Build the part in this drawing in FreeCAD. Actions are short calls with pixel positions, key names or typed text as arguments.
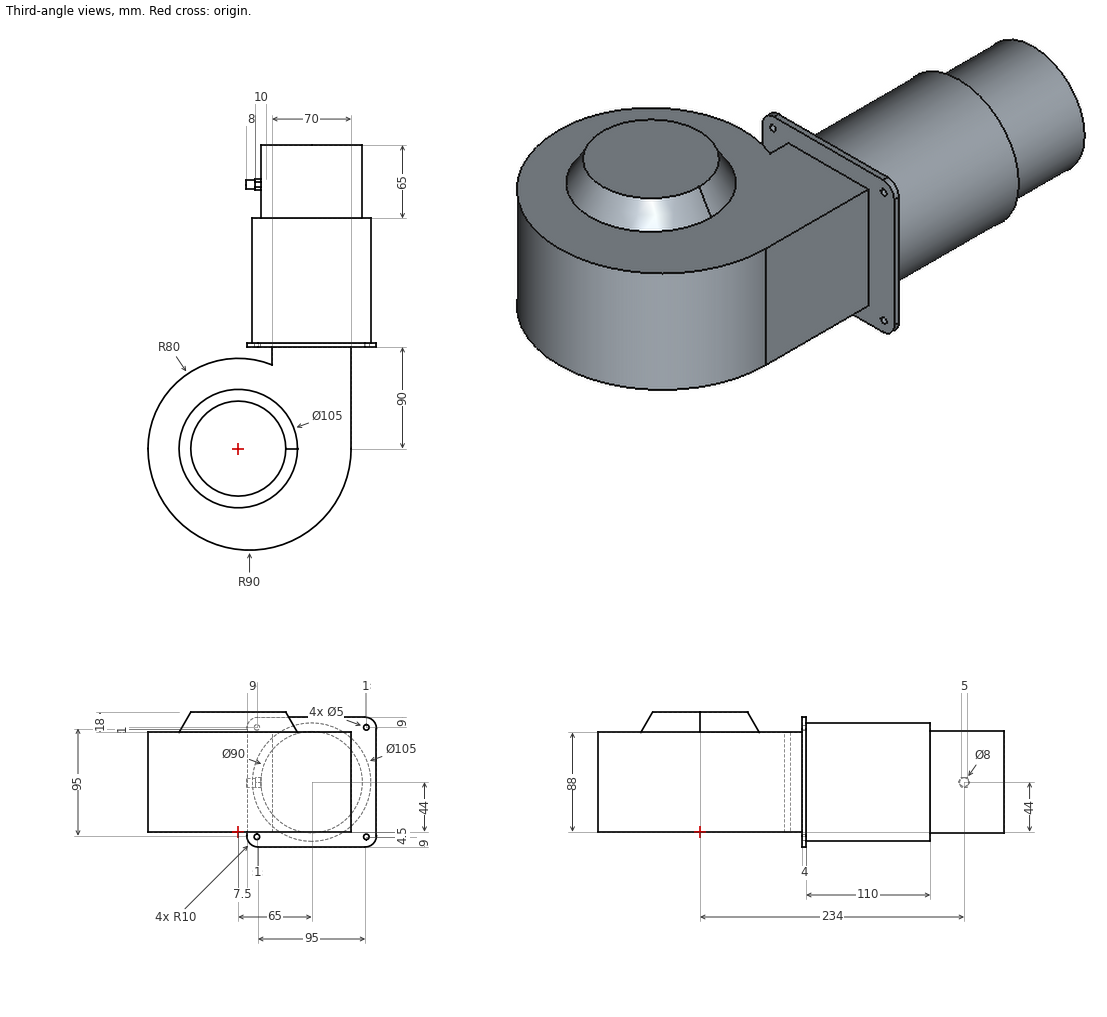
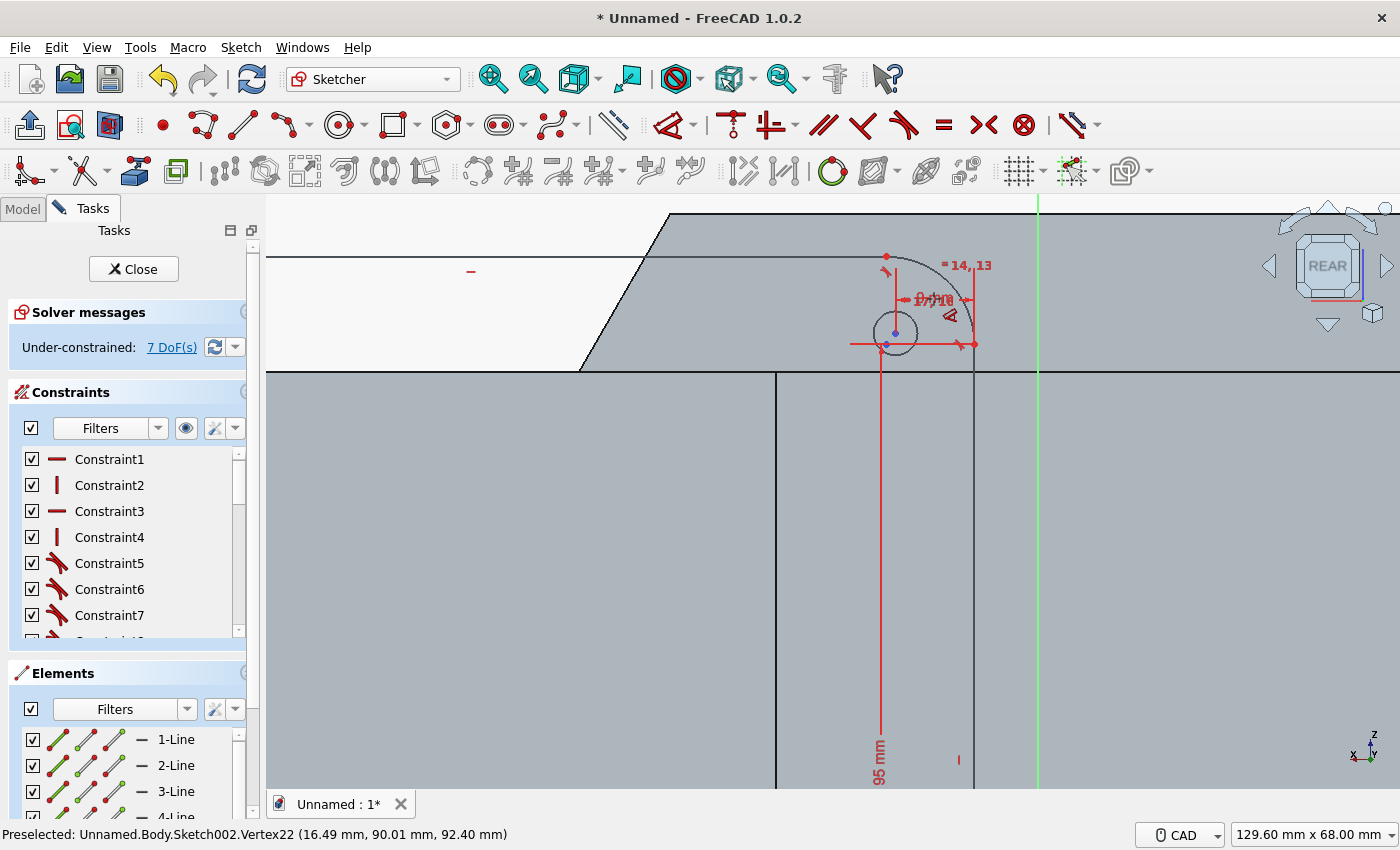
scroll(974, 344, up, 8)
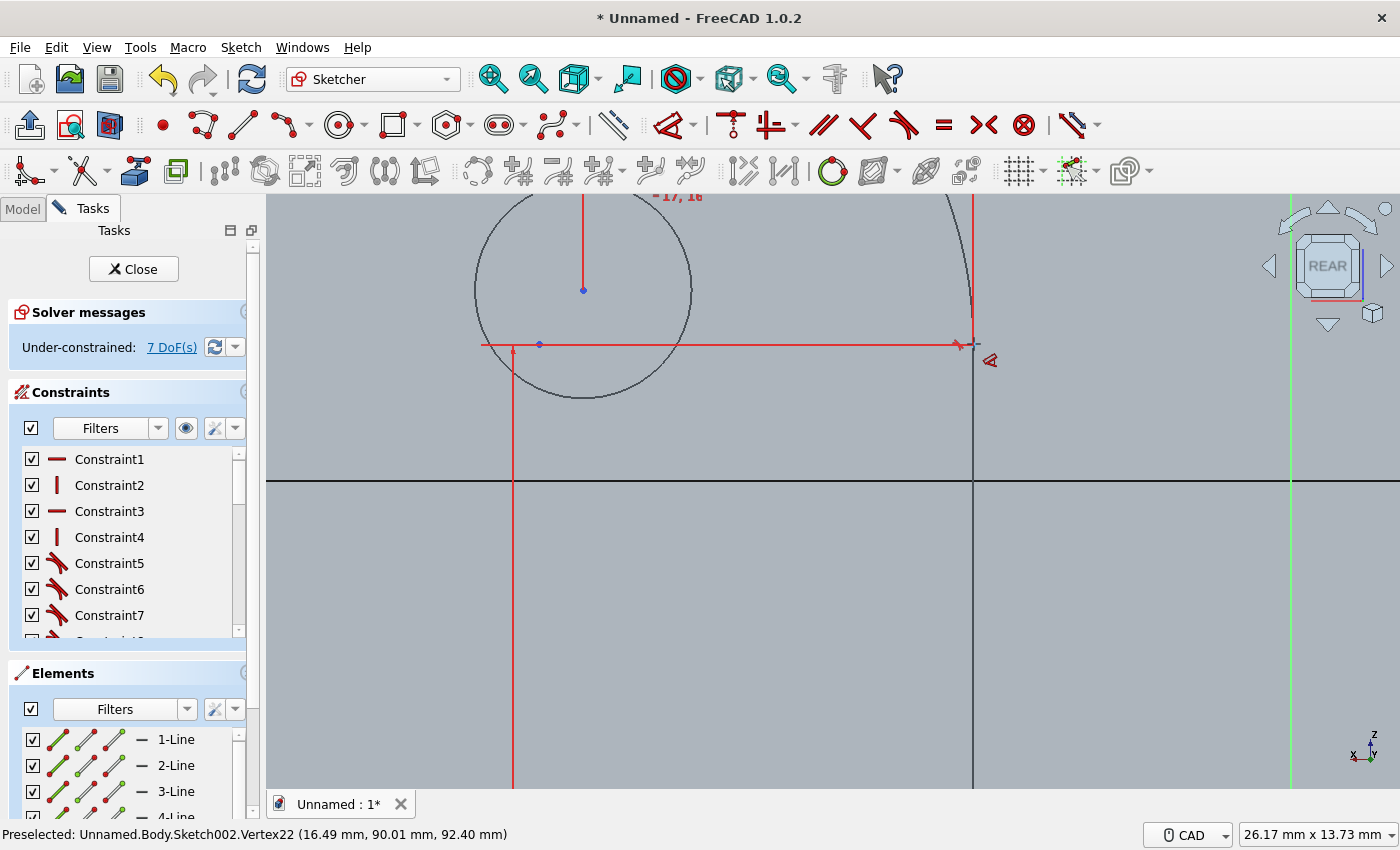
click(973, 345)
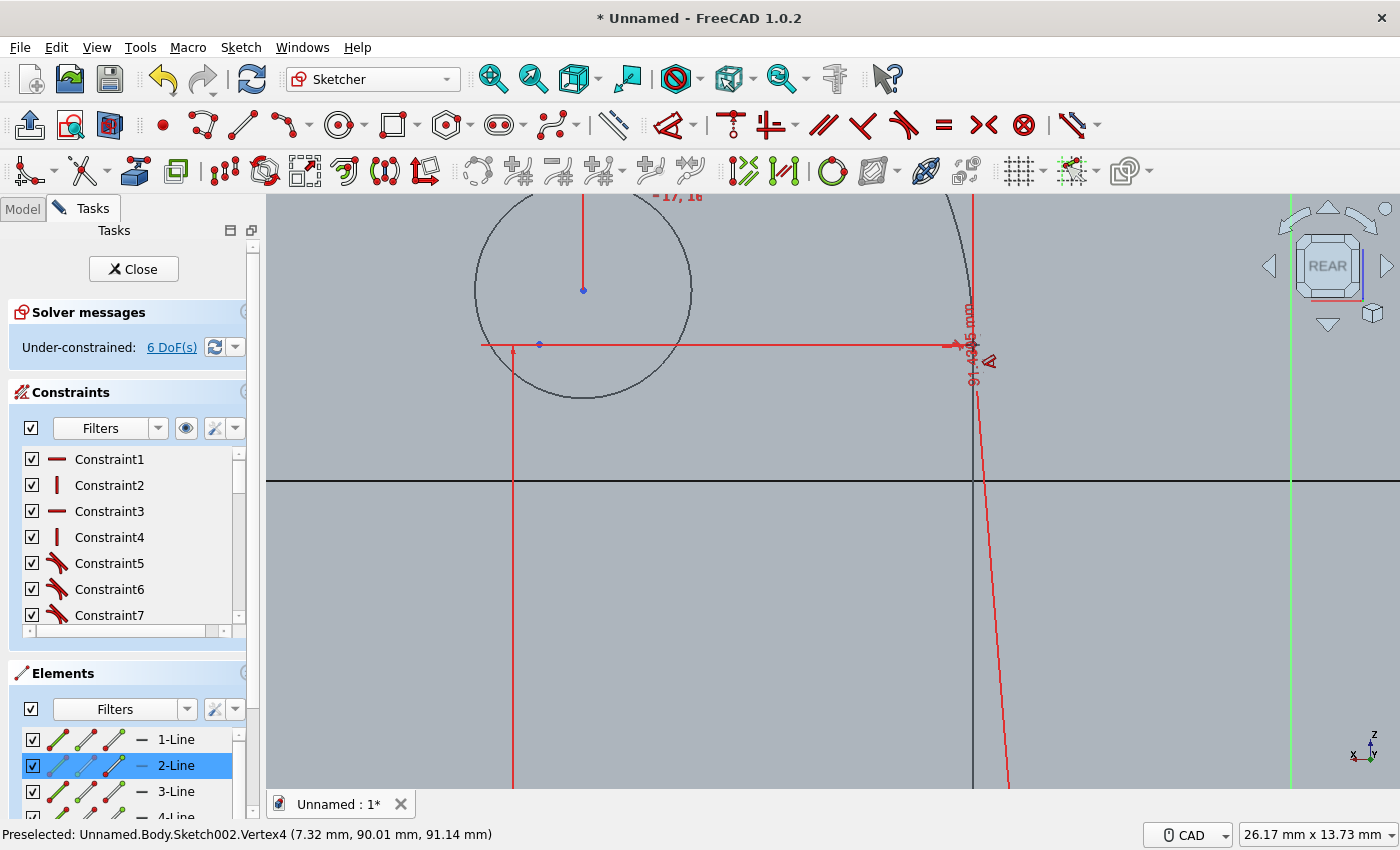
click(583, 290)
click(1007, 317)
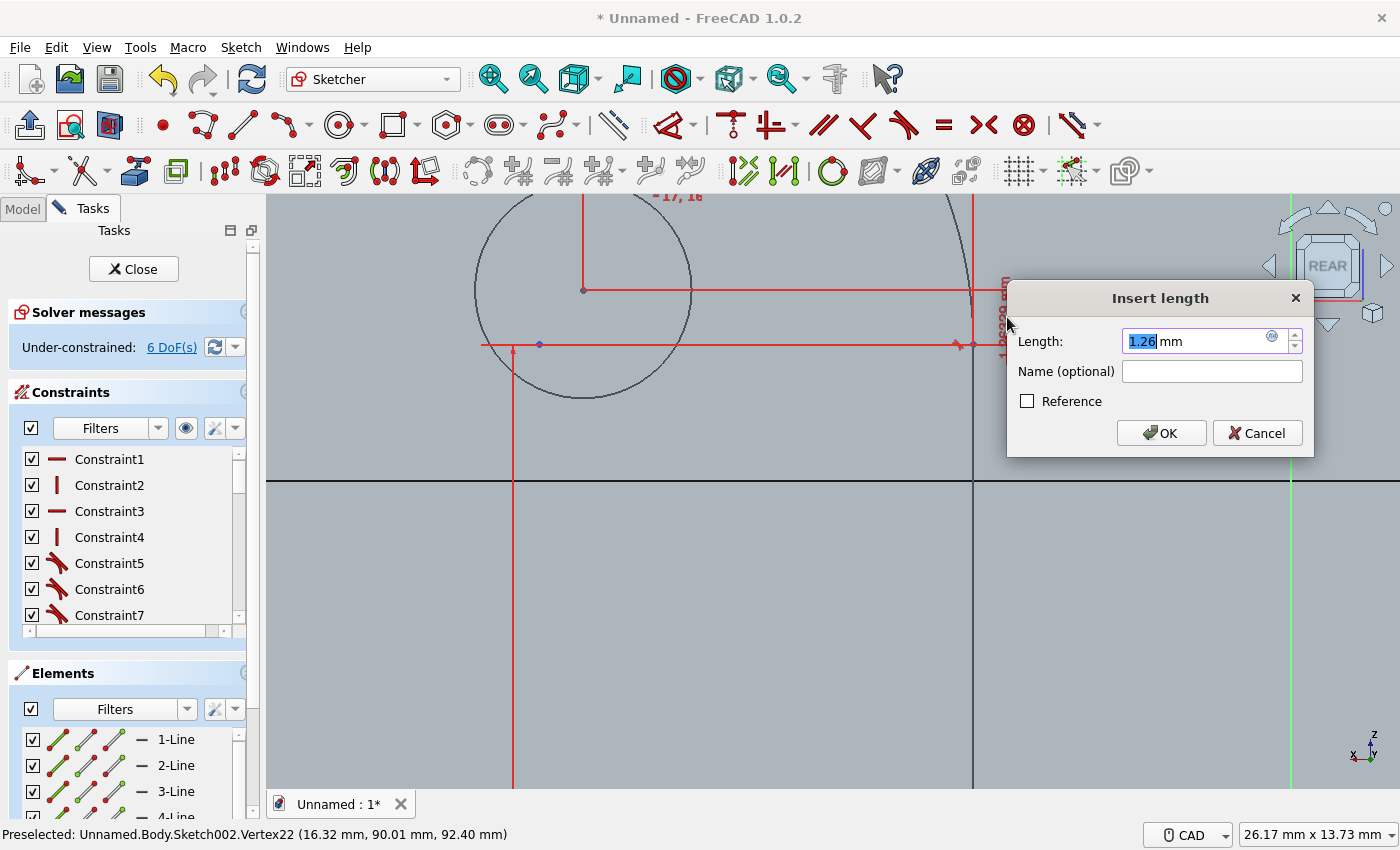
text(1)
key(Return)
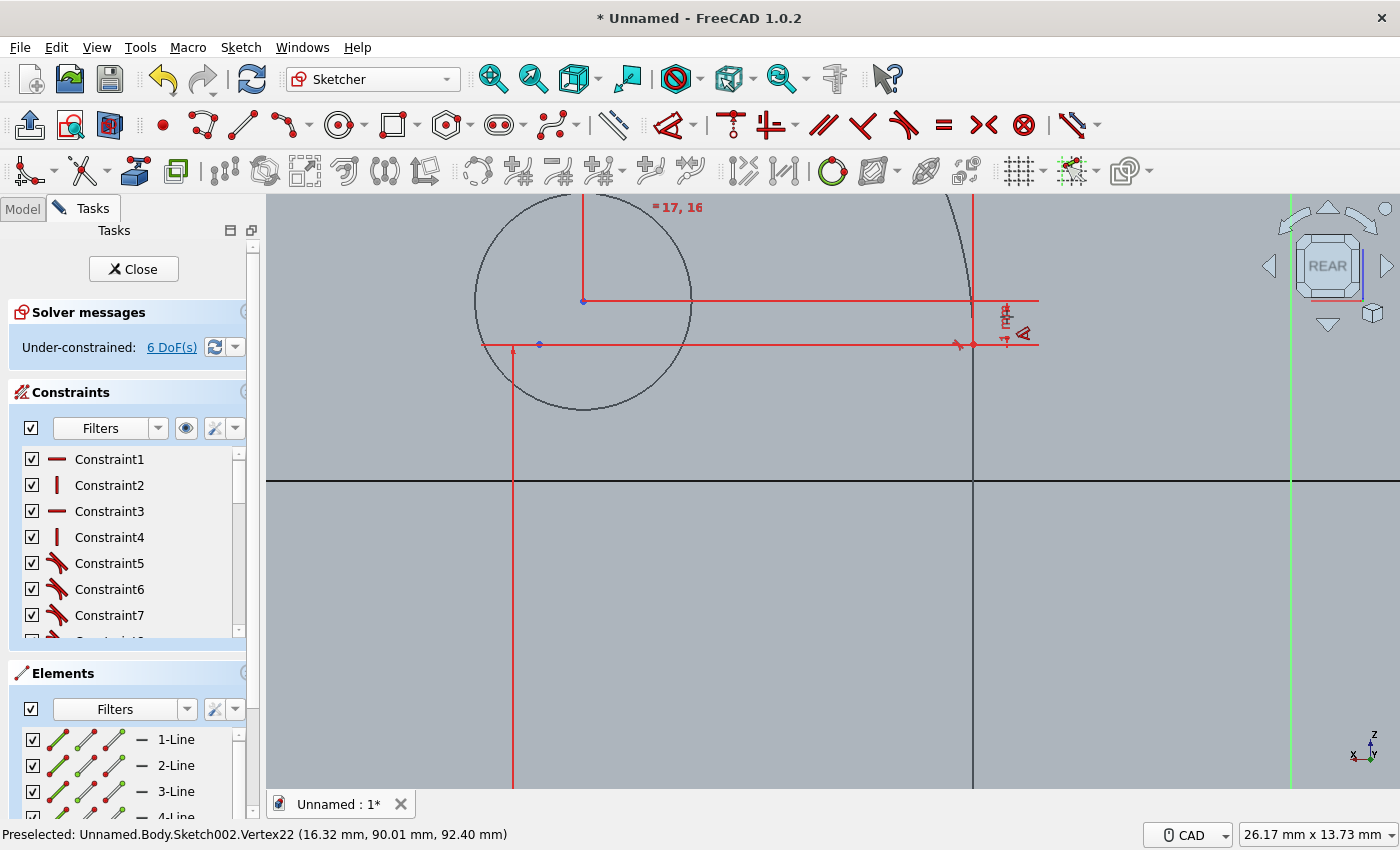
scroll(935, 339, down, 13)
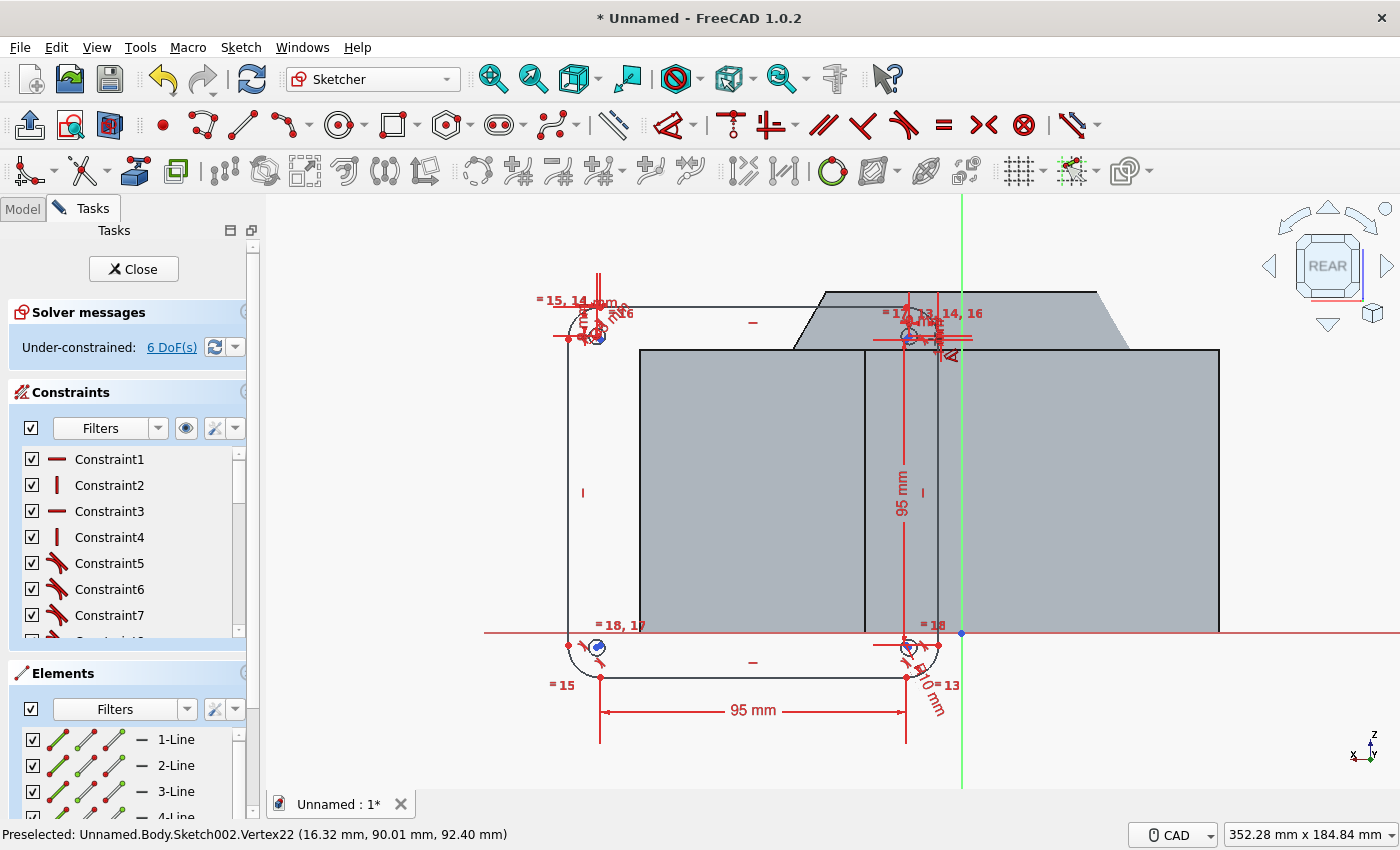
scroll(600, 678, up, 13)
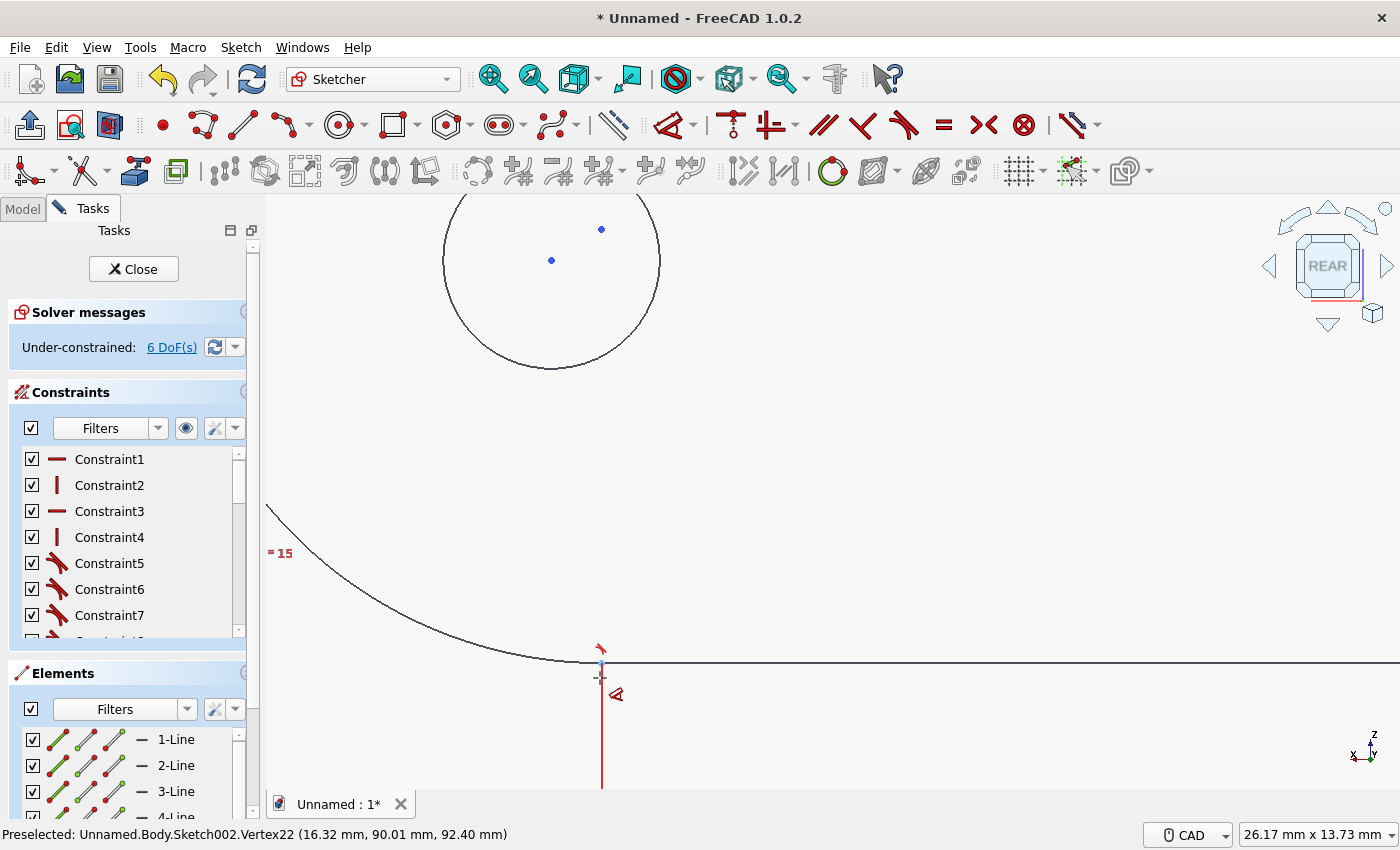
click(602, 663)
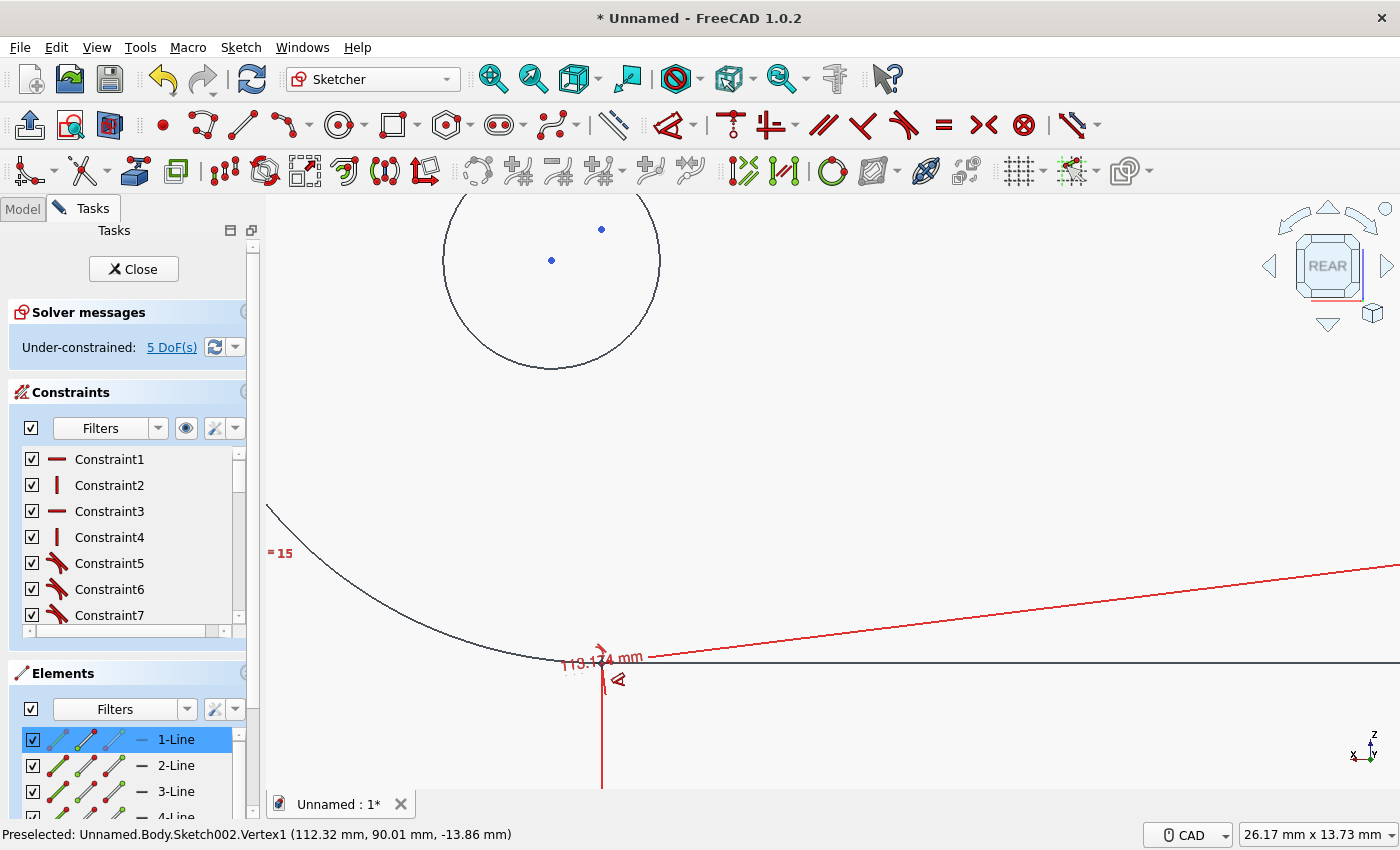
click(552, 260)
click(577, 697)